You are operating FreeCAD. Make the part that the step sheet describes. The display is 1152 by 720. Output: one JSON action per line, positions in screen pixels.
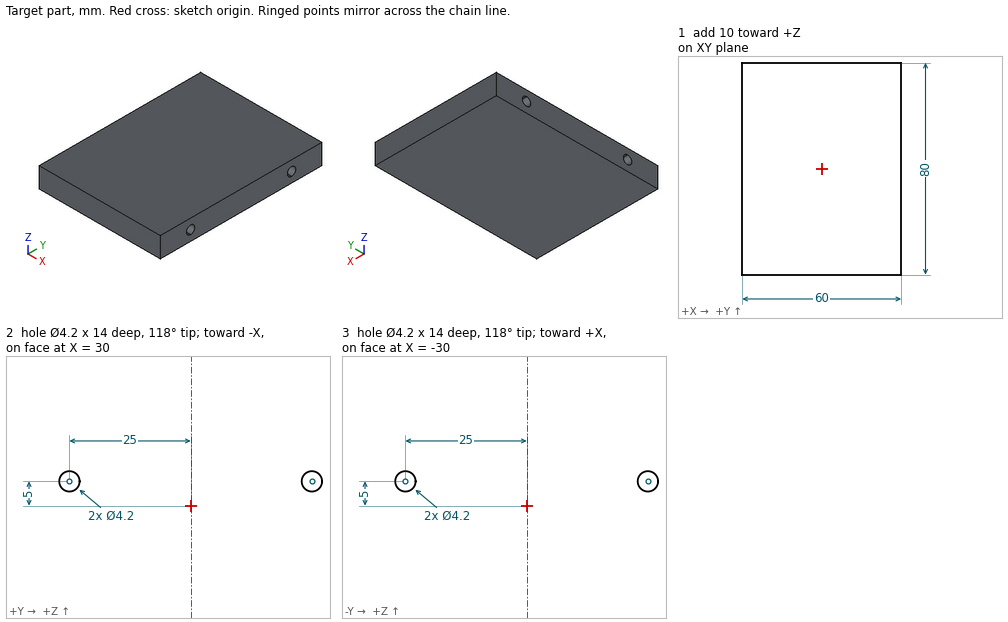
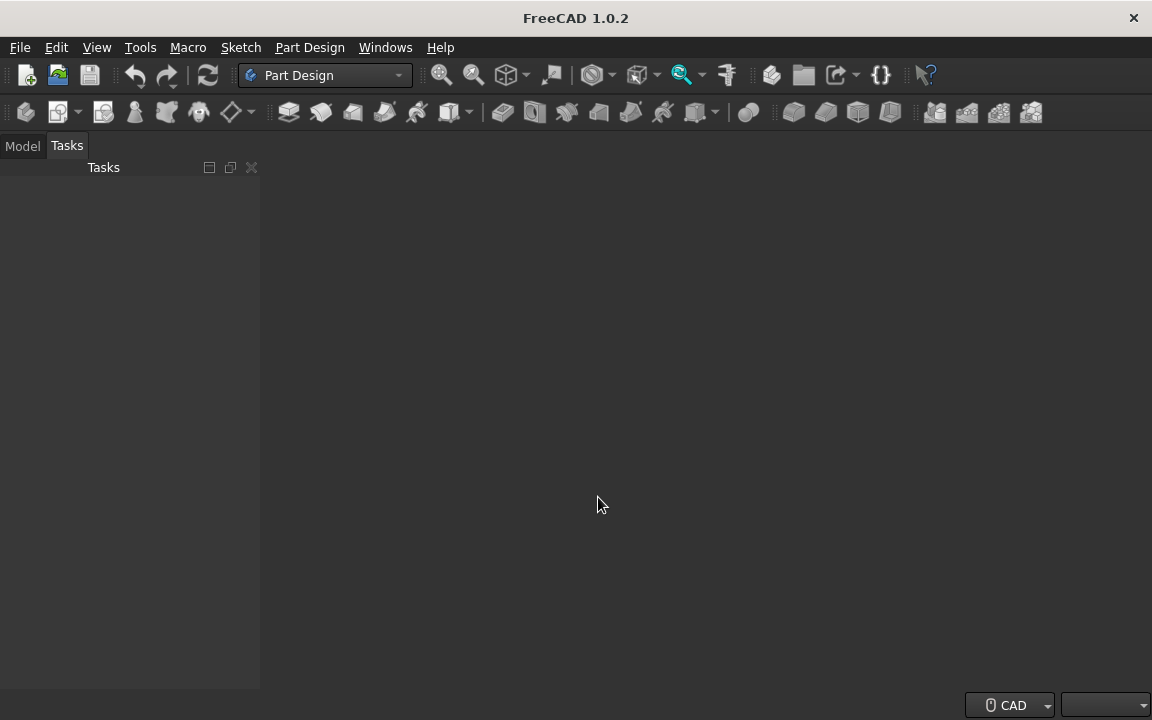
{"action": "left_click", "coordinate": [26, 76]}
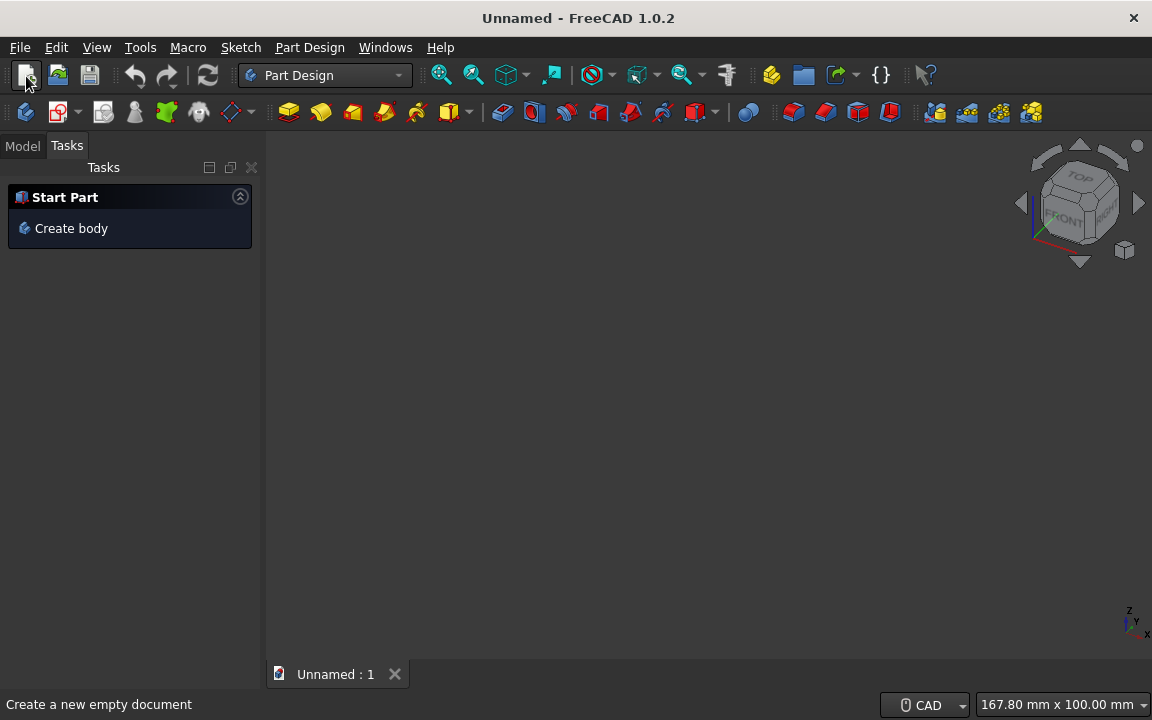
{"action": "left_click", "coordinate": [58, 112]}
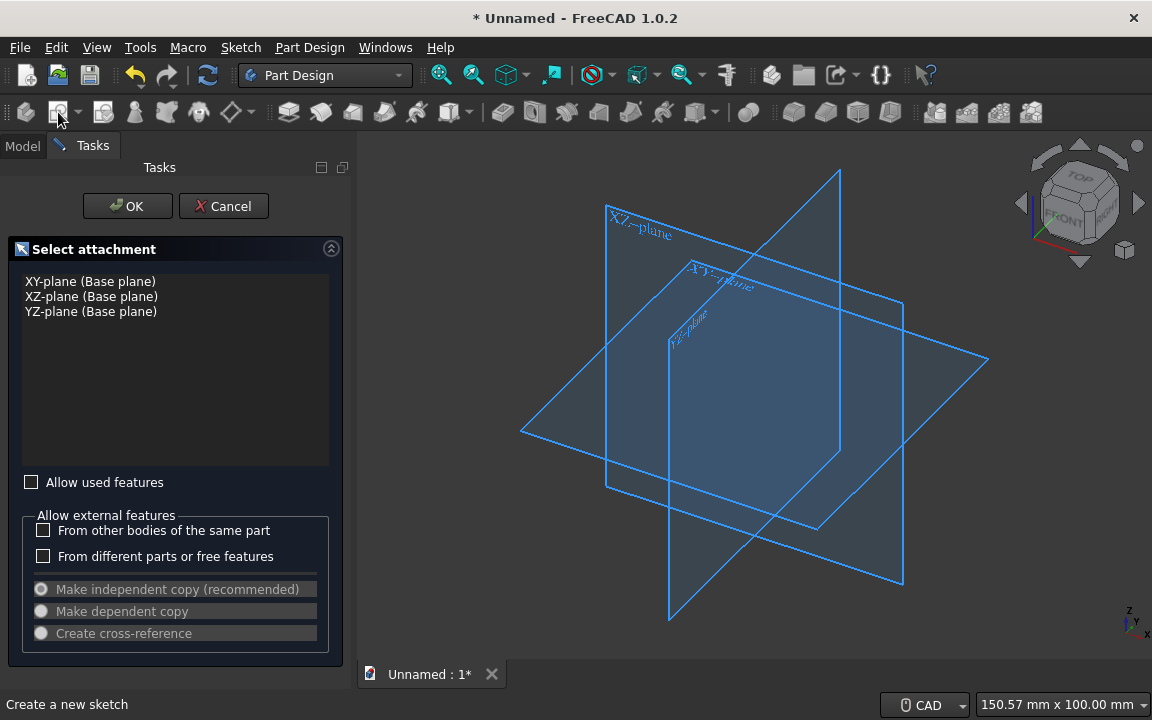
{"action": "left_click", "coordinate": [82, 282]}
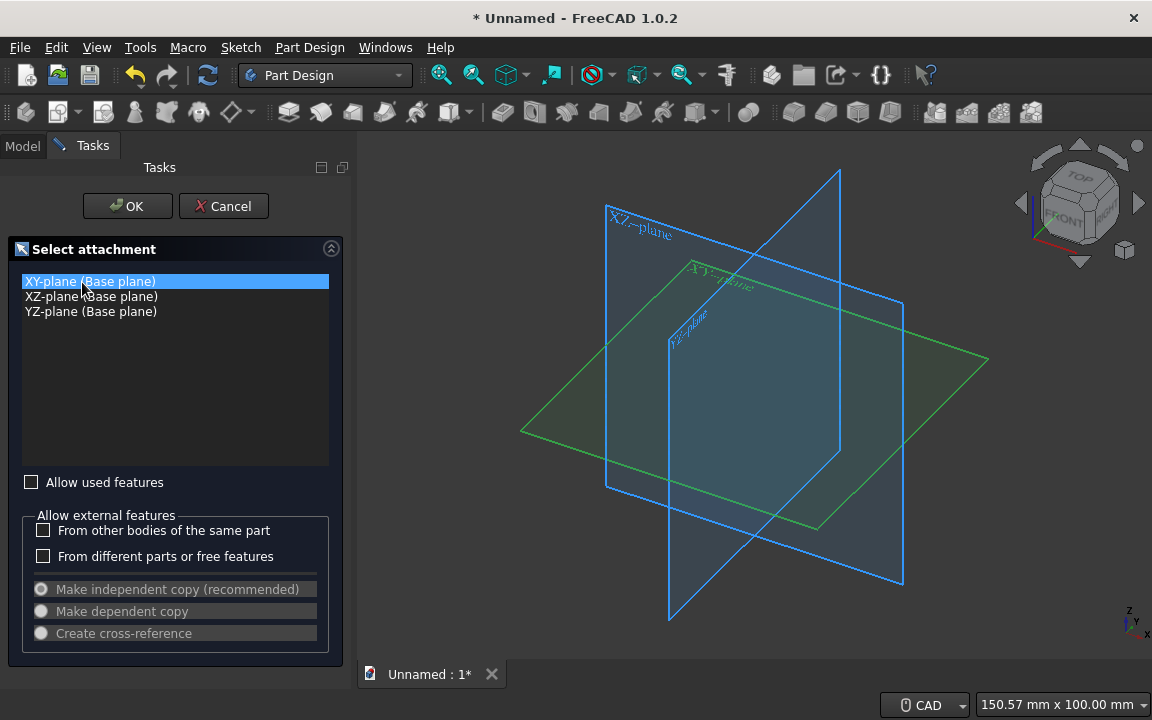
{"action": "left_click", "coordinate": [128, 206]}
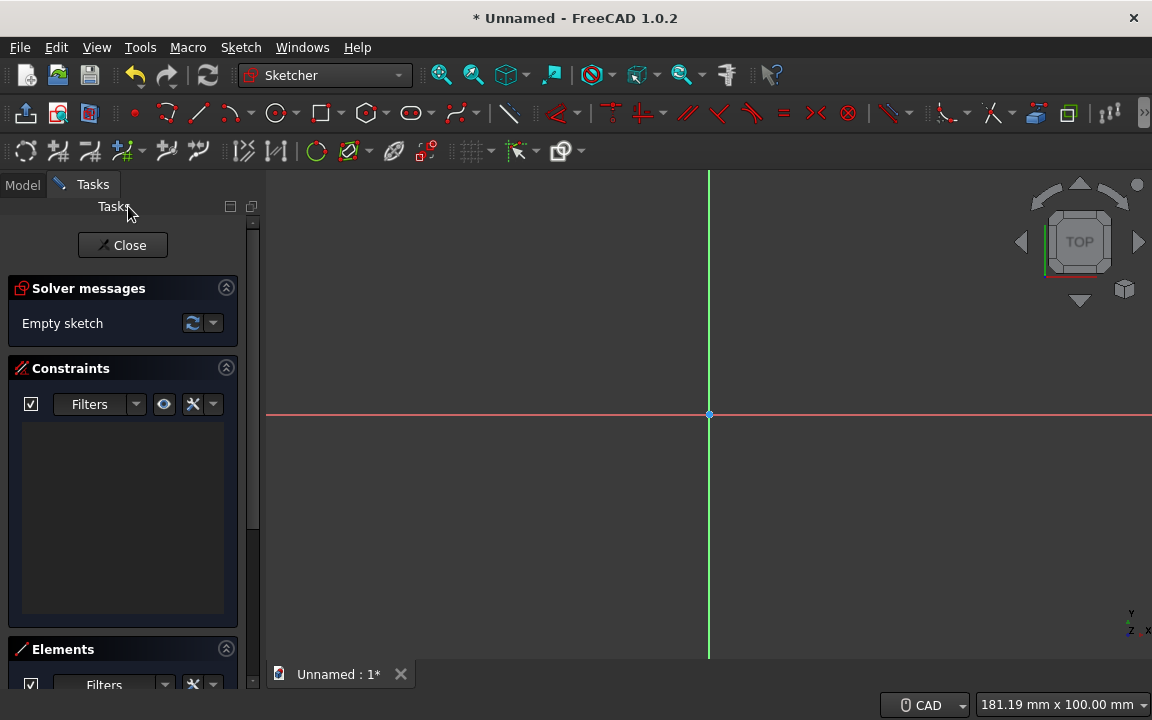
{"action": "scroll", "coordinate": [331, 415], "scroll_direction": "down", "scroll_amount": 1}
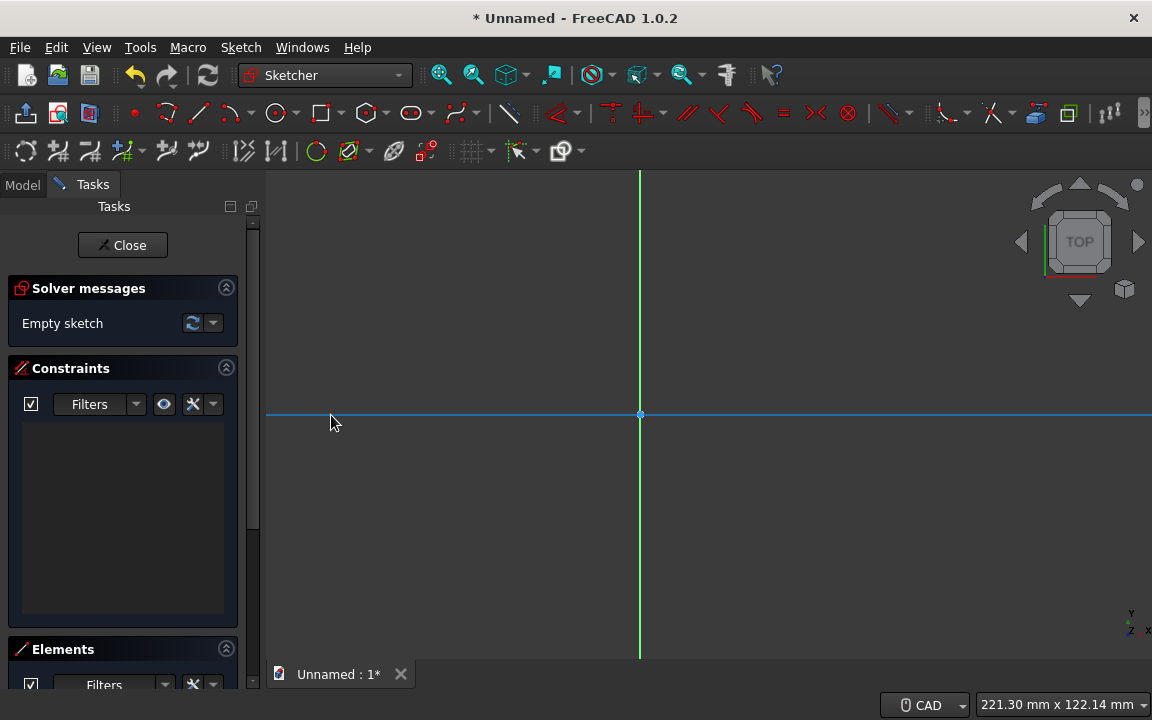
{"action": "key", "text": "g v"}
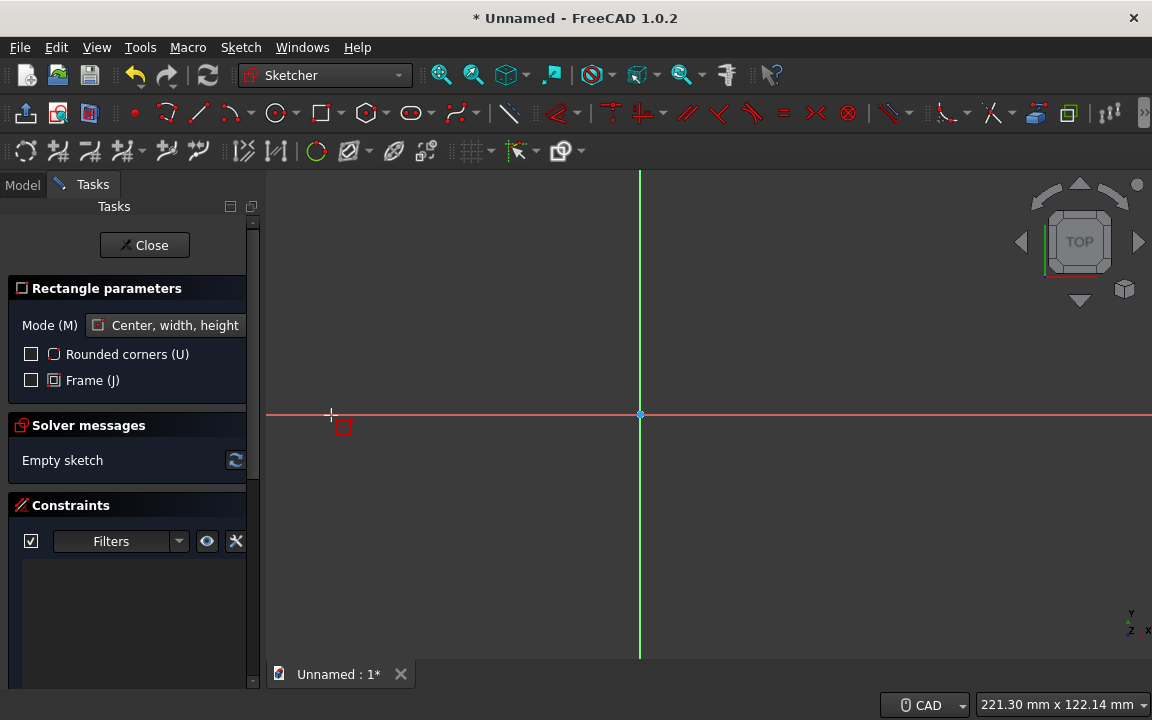
{"action": "left_click", "coordinate": [640, 415]}
{"action": "mouse_move", "coordinate": [761, 255]}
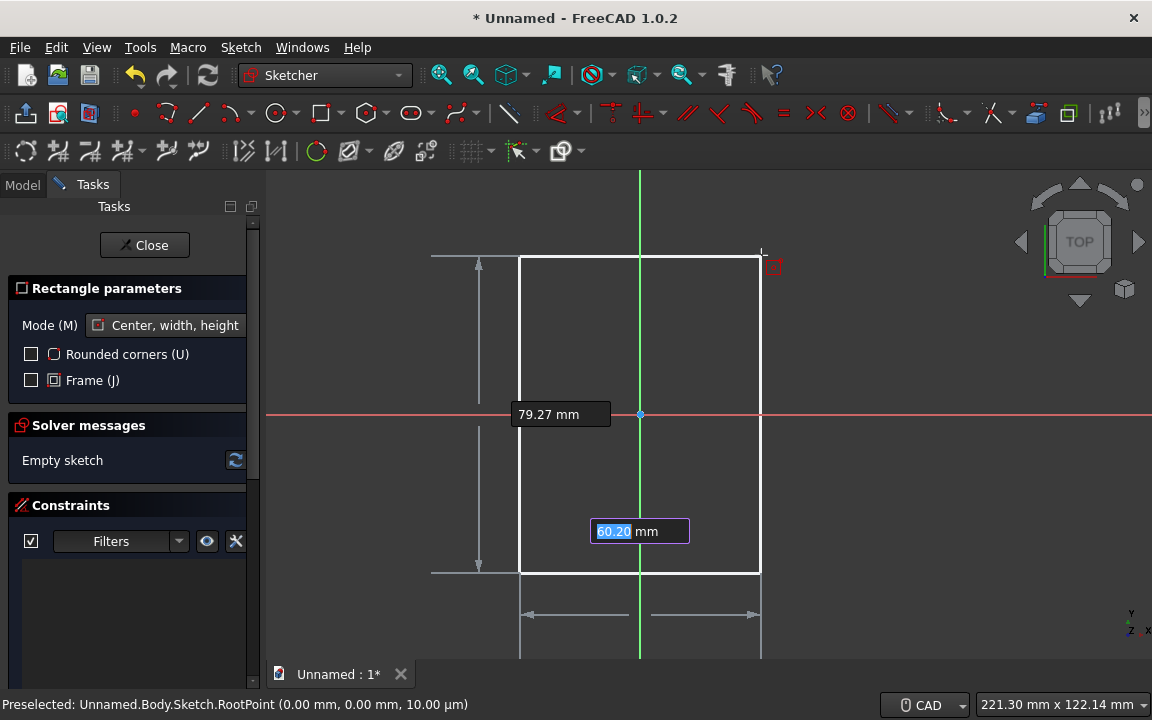
{"action": "type", "text": "60"}
{"action": "key", "text": "Tab"}
{"action": "type", "text": "80"}
{"action": "key", "text": "Return"}
{"action": "key", "text": "Escape"}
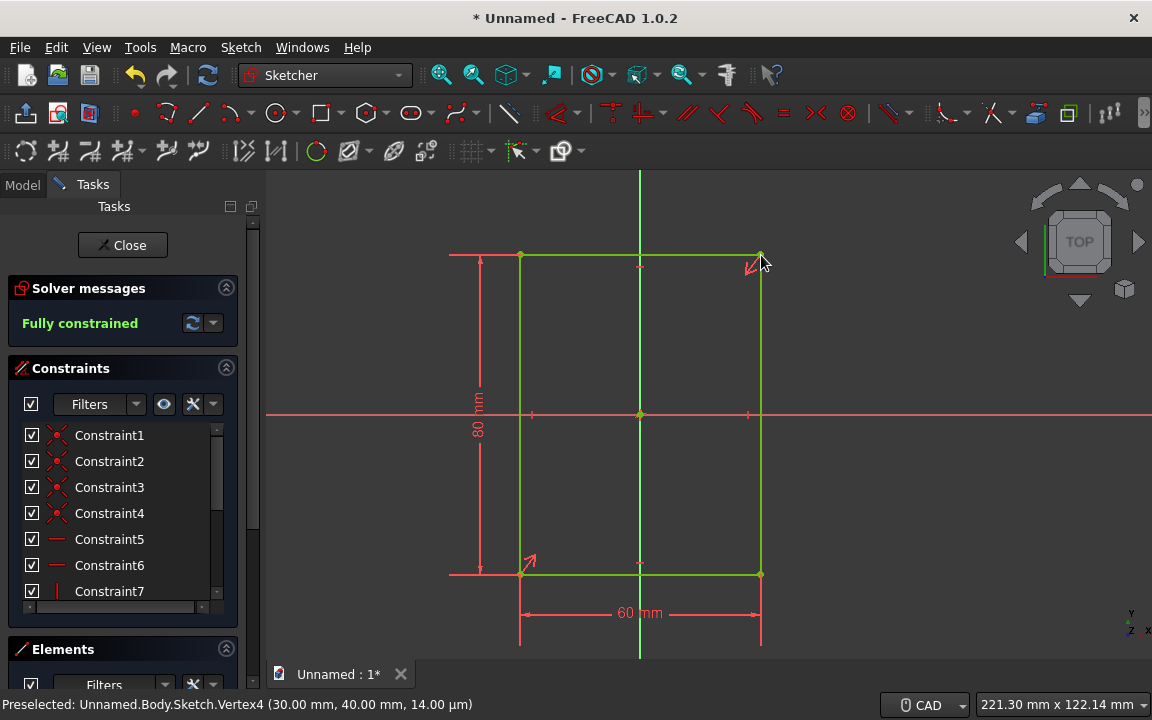
{"action": "left_click", "coordinate": [123, 245]}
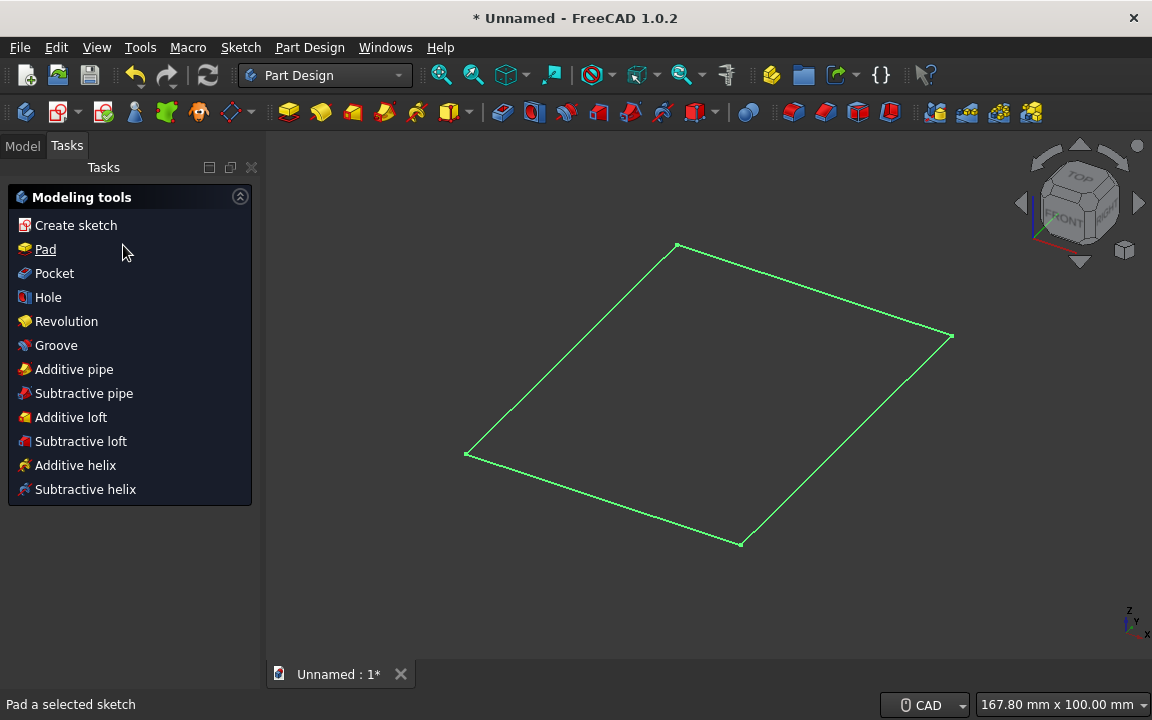
{"action": "left_click", "coordinate": [290, 112]}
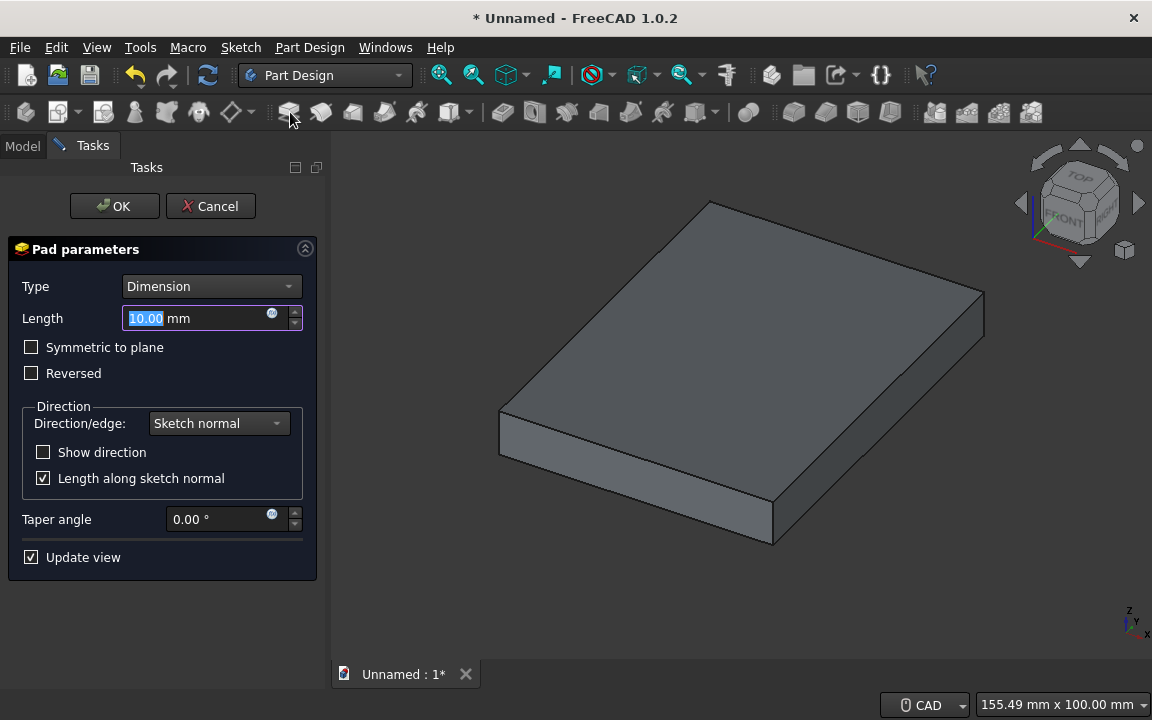
{"action": "type", "text": "10"}
{"action": "key", "text": "Tab"}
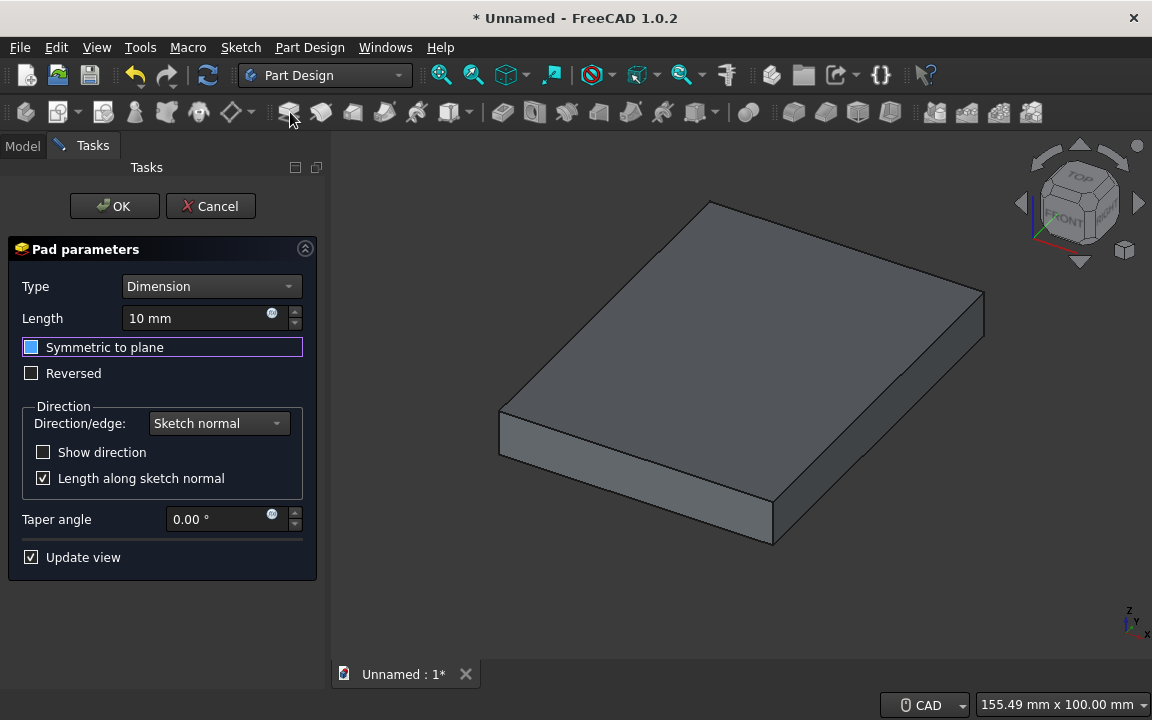
{"action": "left_click", "coordinate": [115, 206]}